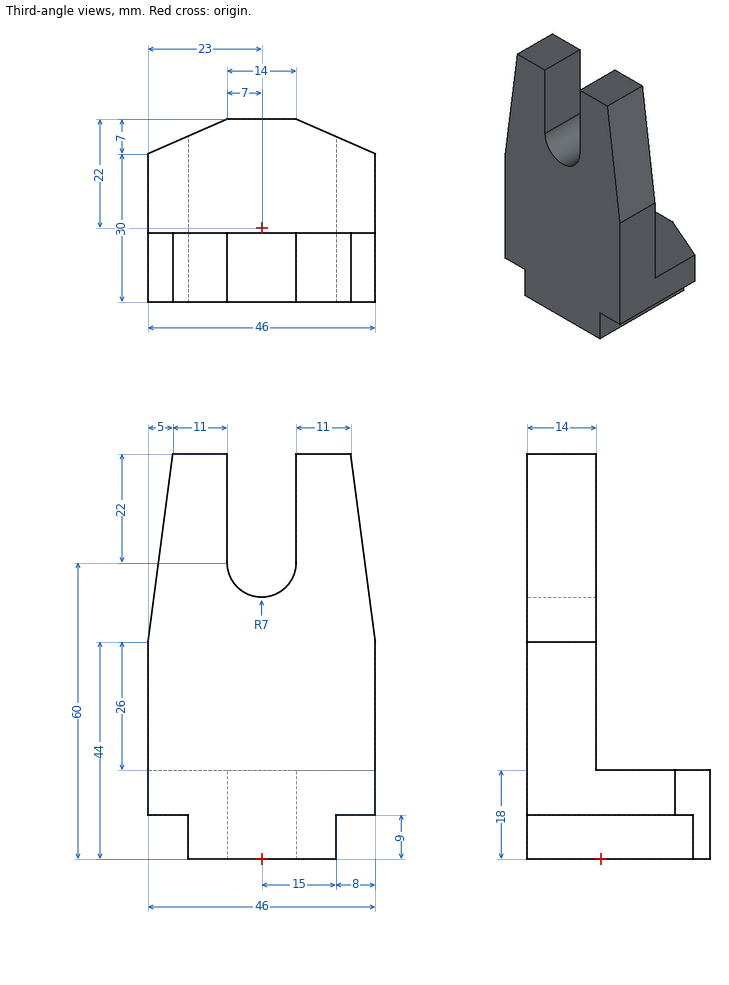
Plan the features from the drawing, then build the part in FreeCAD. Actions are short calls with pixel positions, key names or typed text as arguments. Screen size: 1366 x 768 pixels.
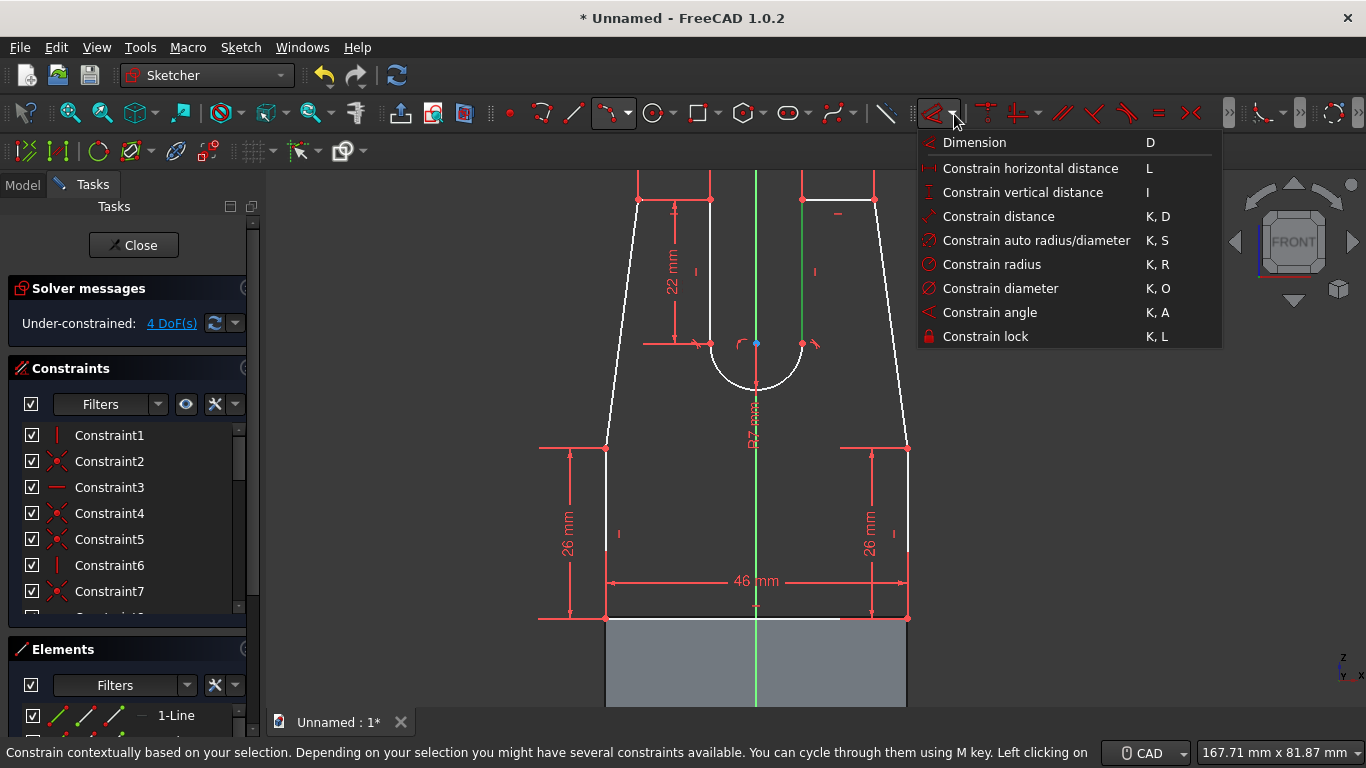
click(1070, 192)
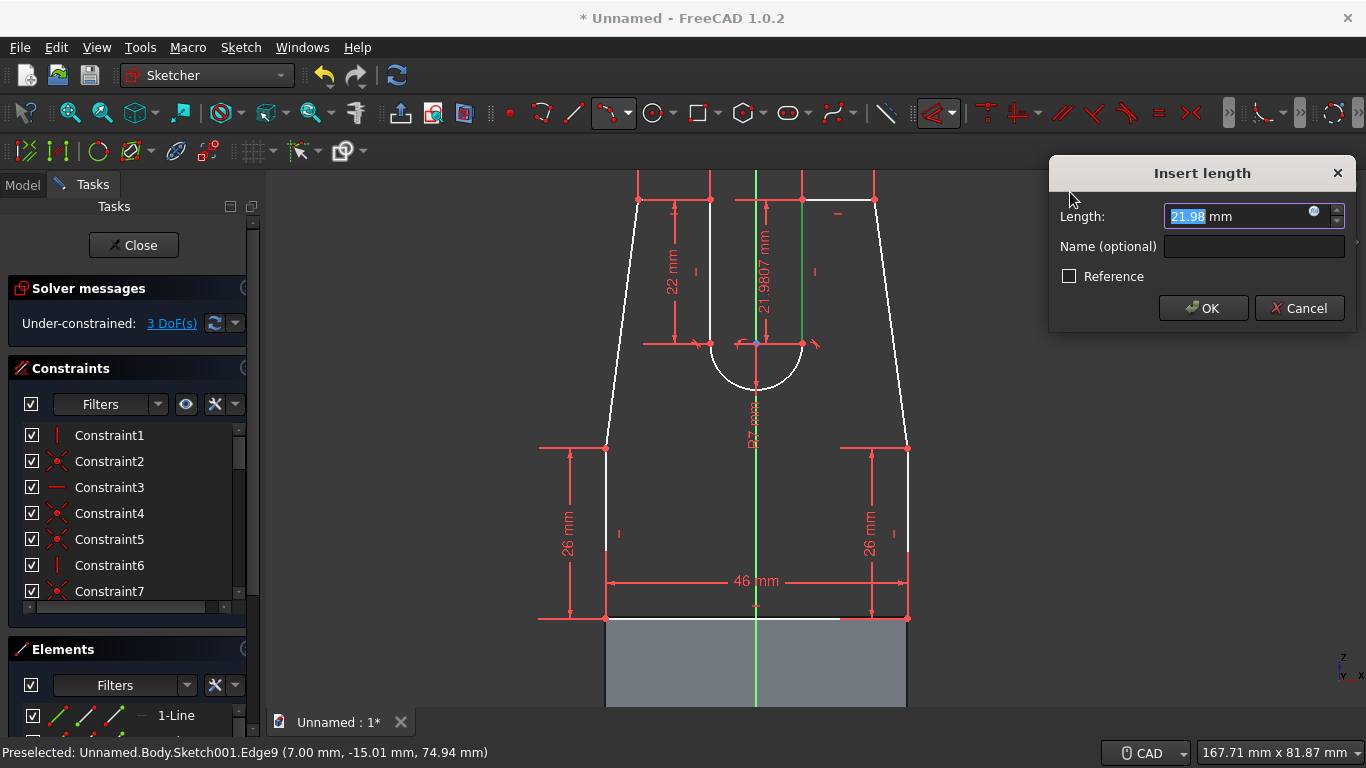
text(22)
key(Return)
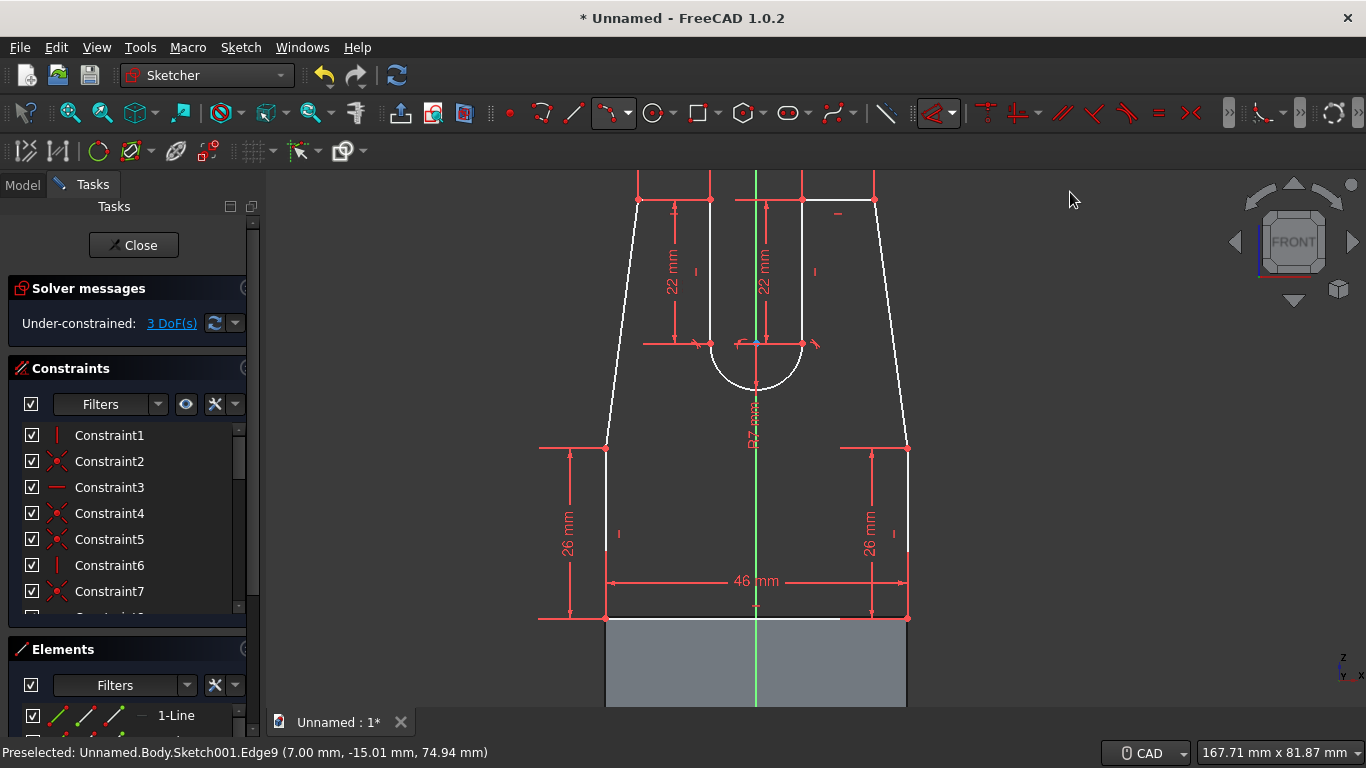
click(629, 274)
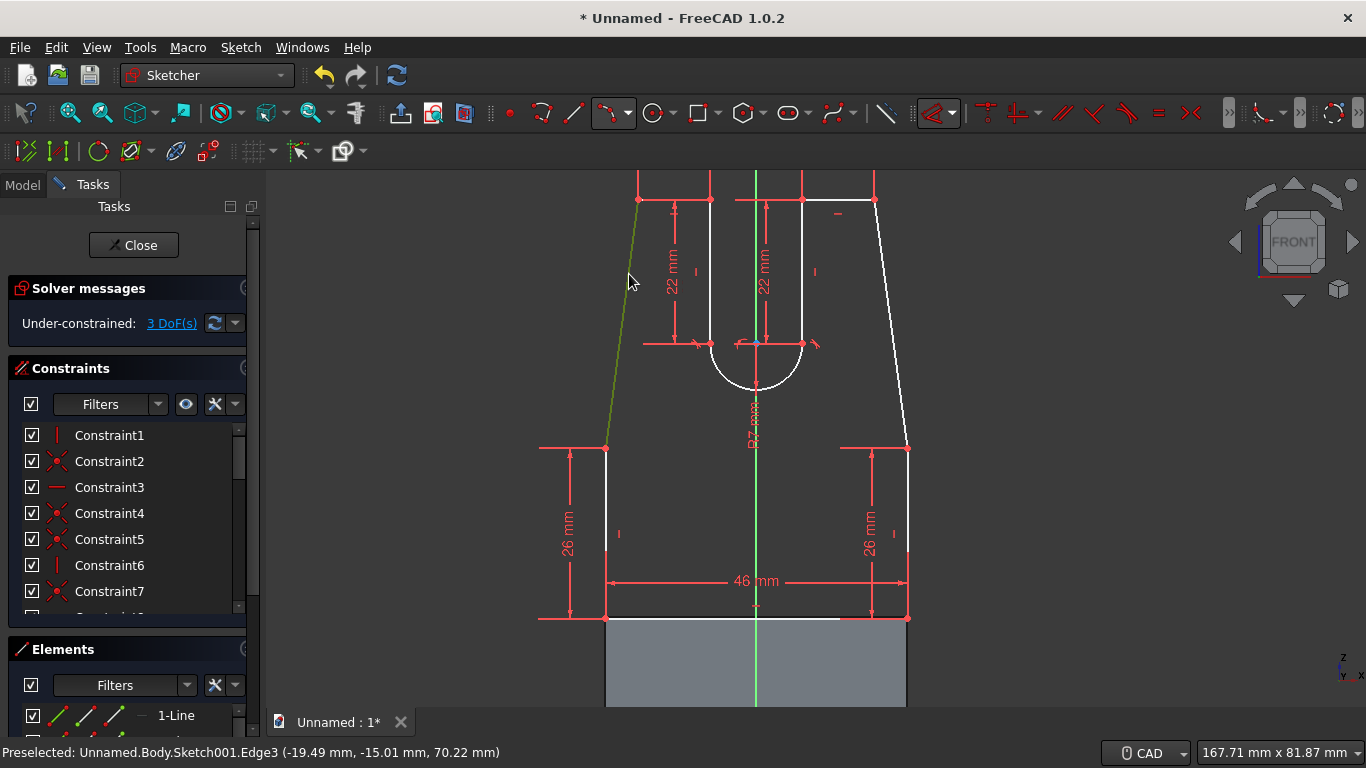
click(954, 114)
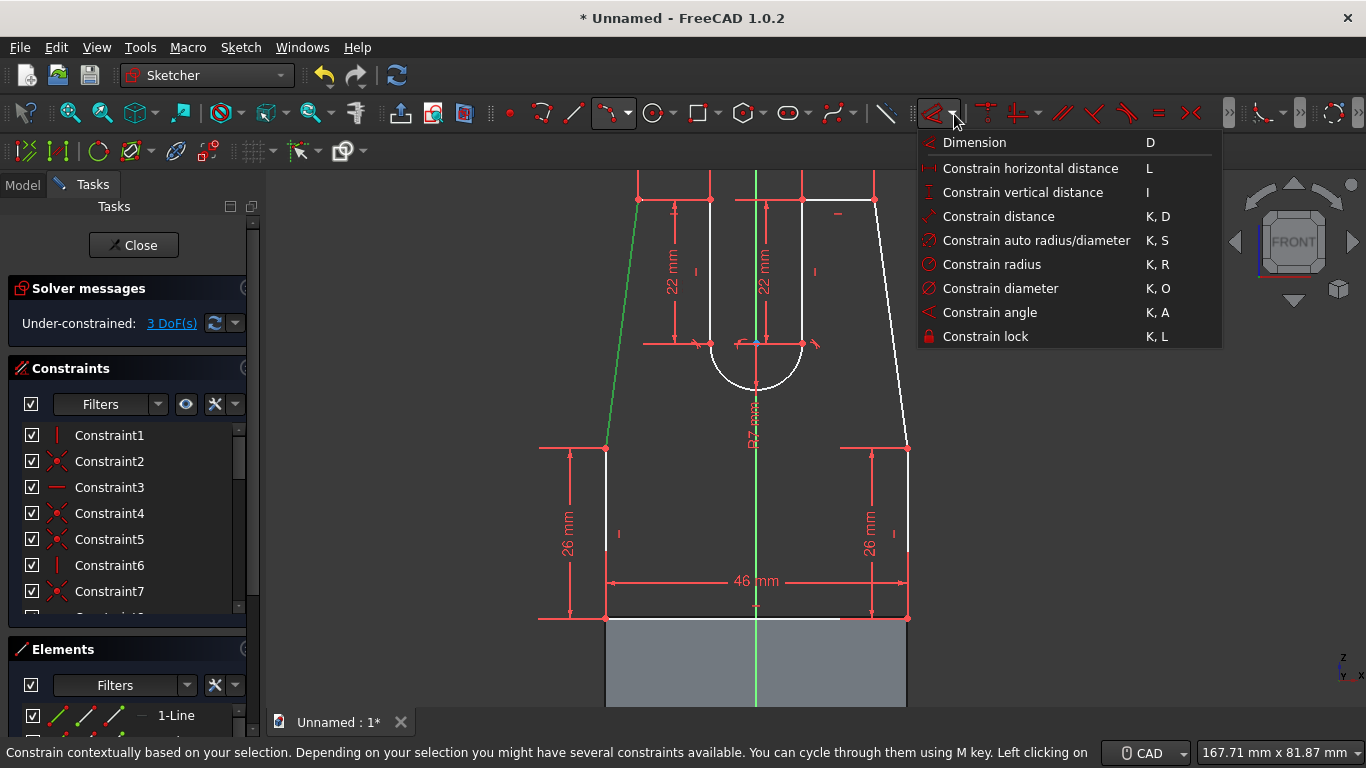
click(1070, 168)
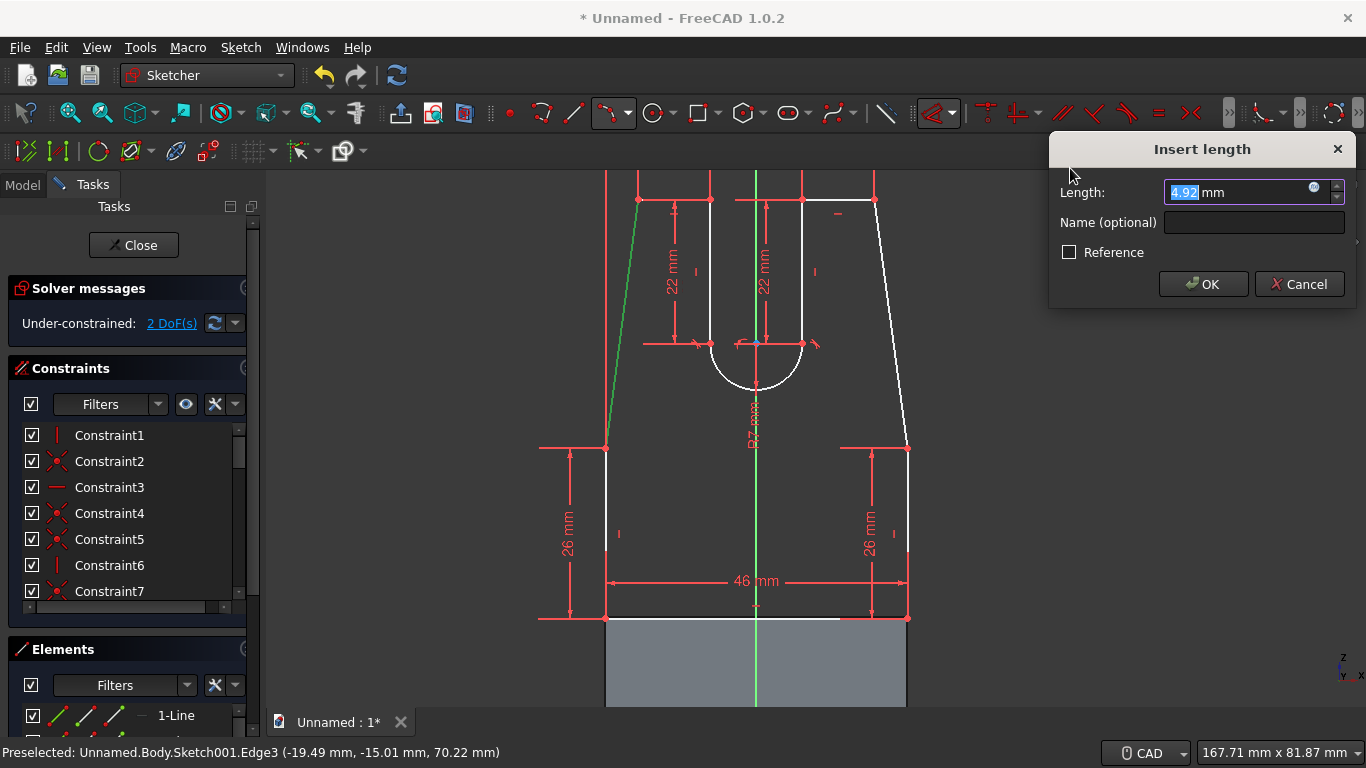
text(5)
key(Return)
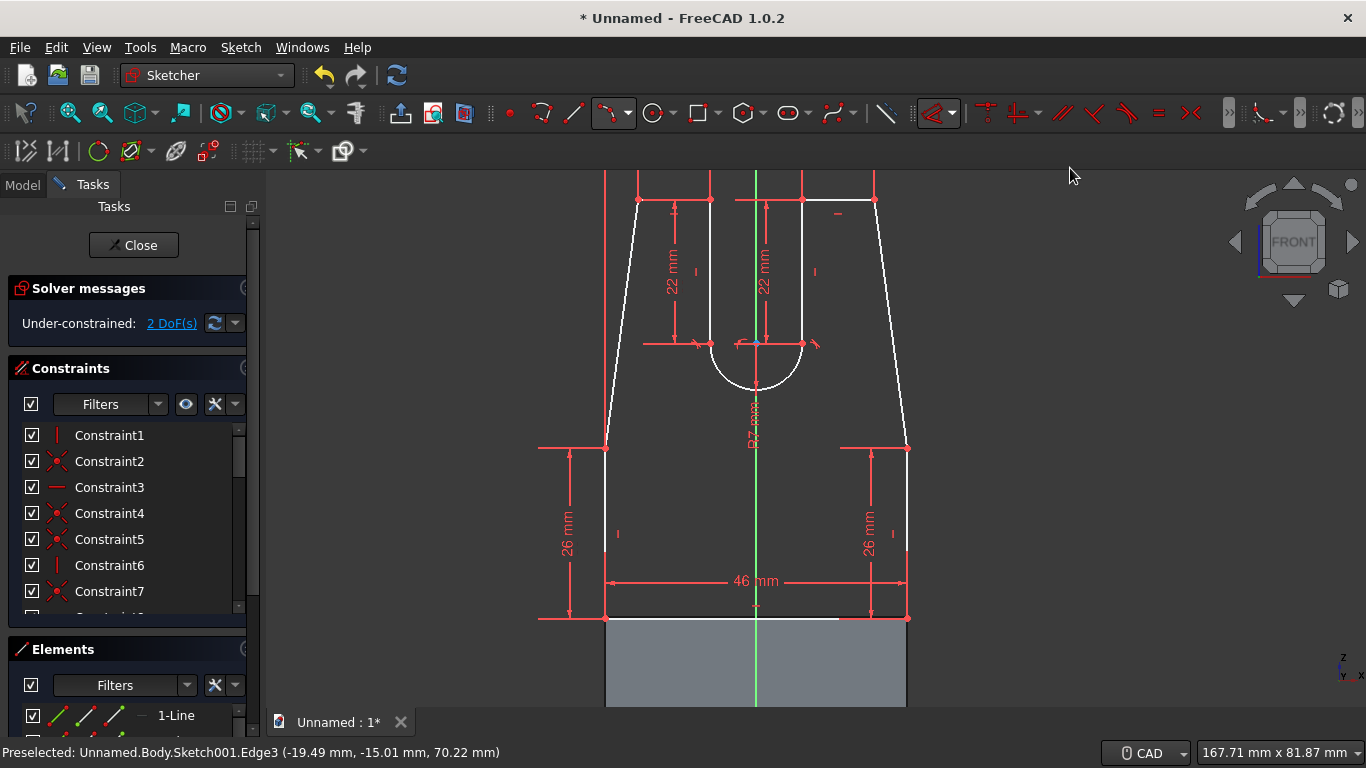
click(710, 344)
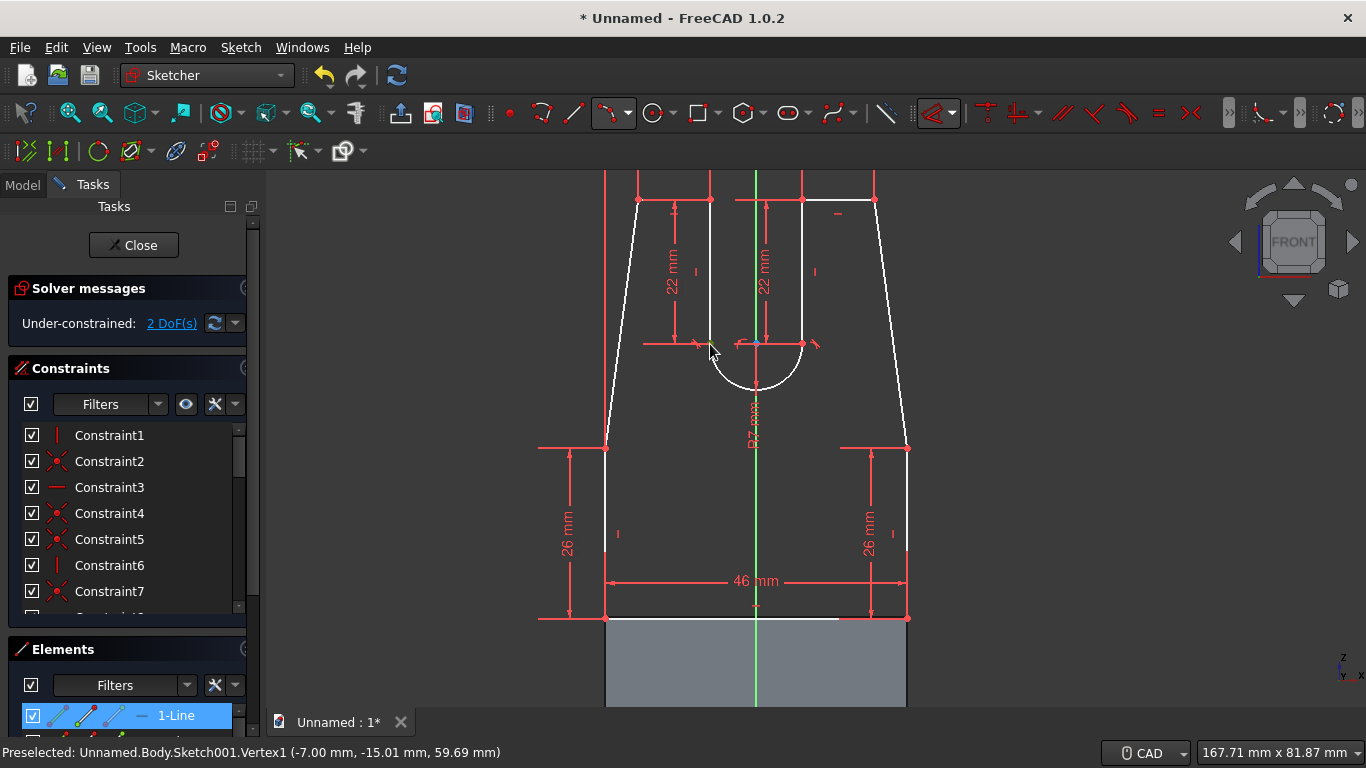
click(954, 114)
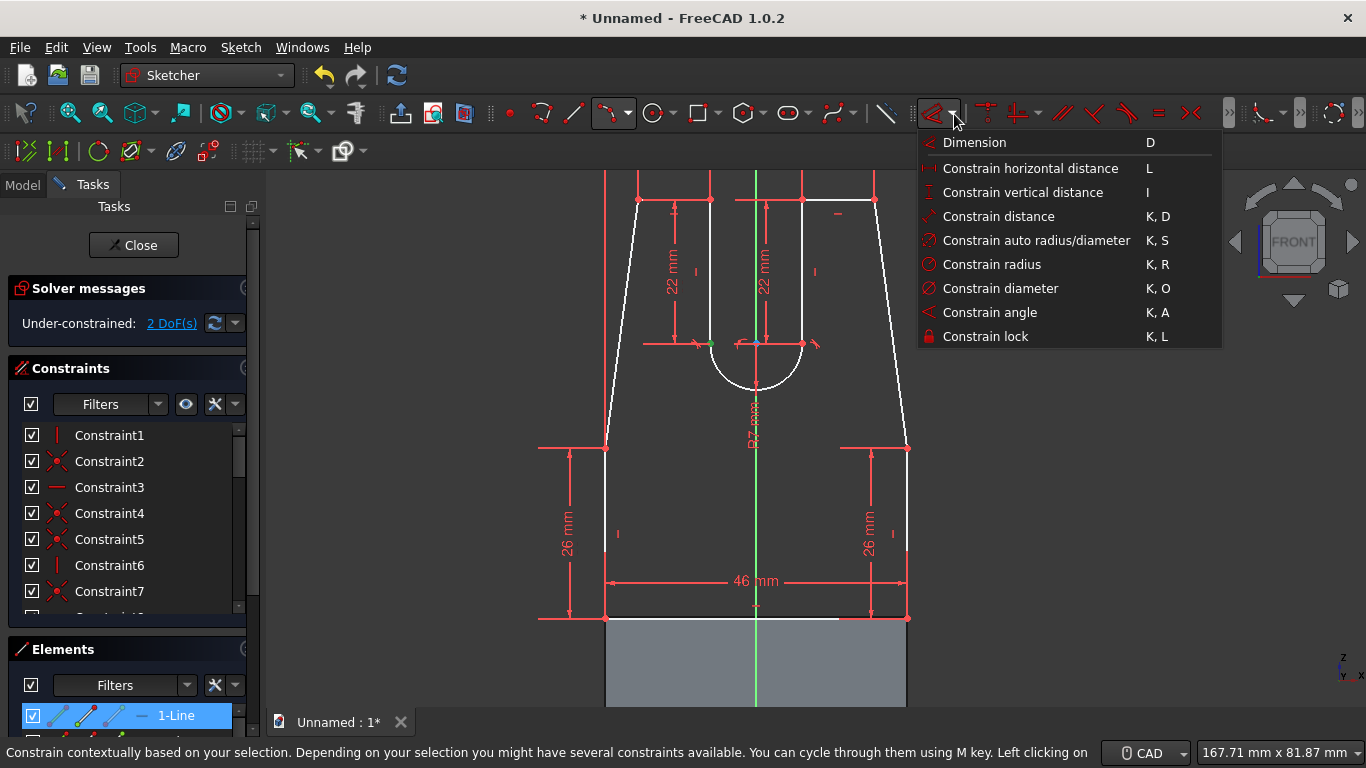
click(1070, 192)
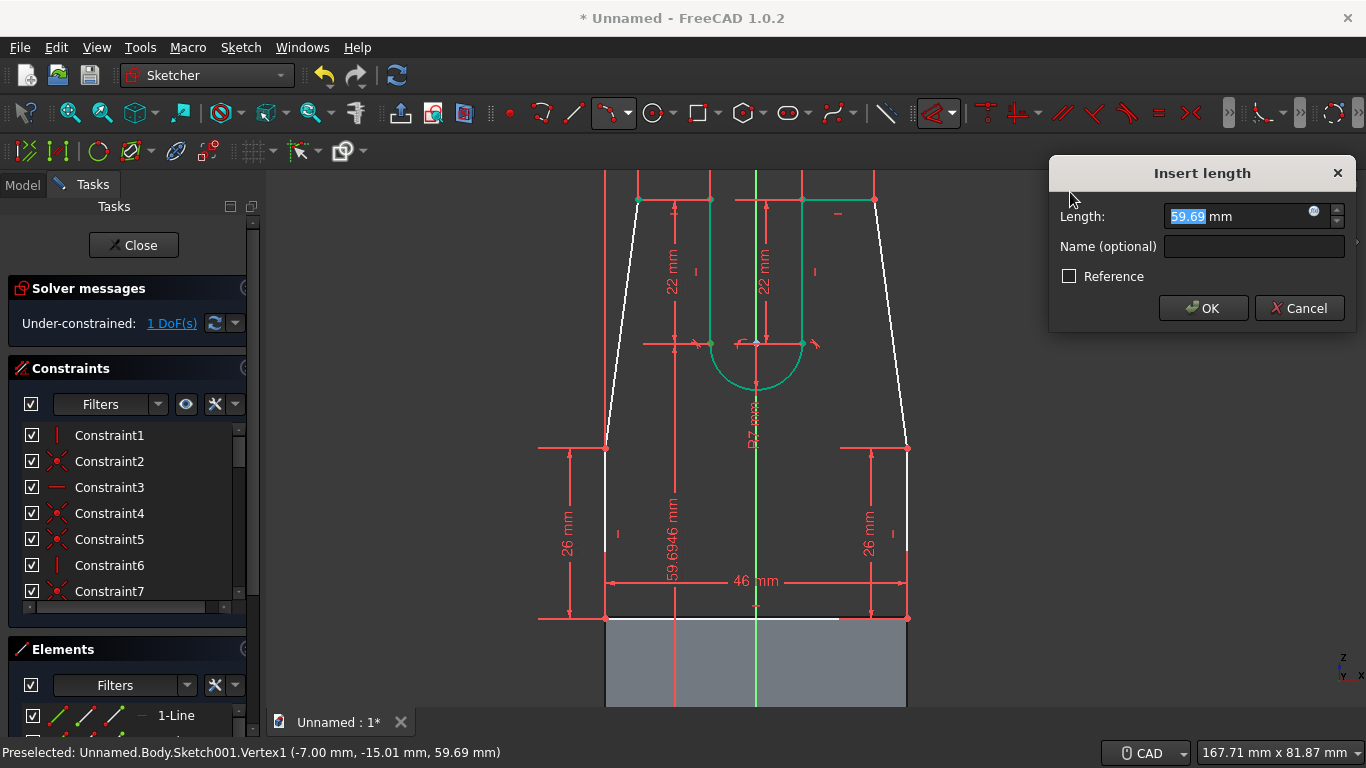
text(60)
key(Return)